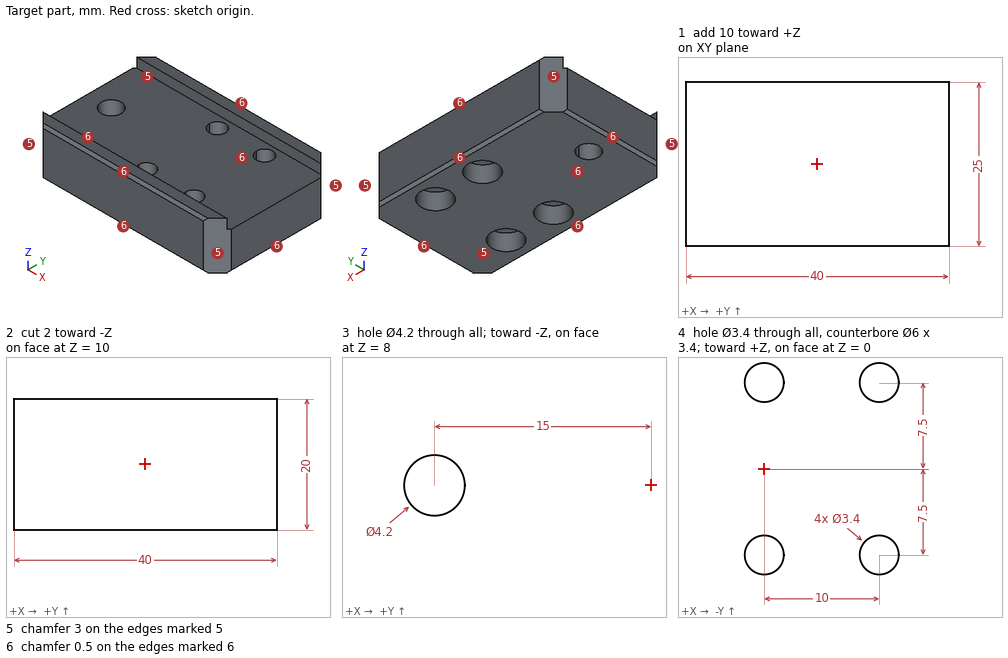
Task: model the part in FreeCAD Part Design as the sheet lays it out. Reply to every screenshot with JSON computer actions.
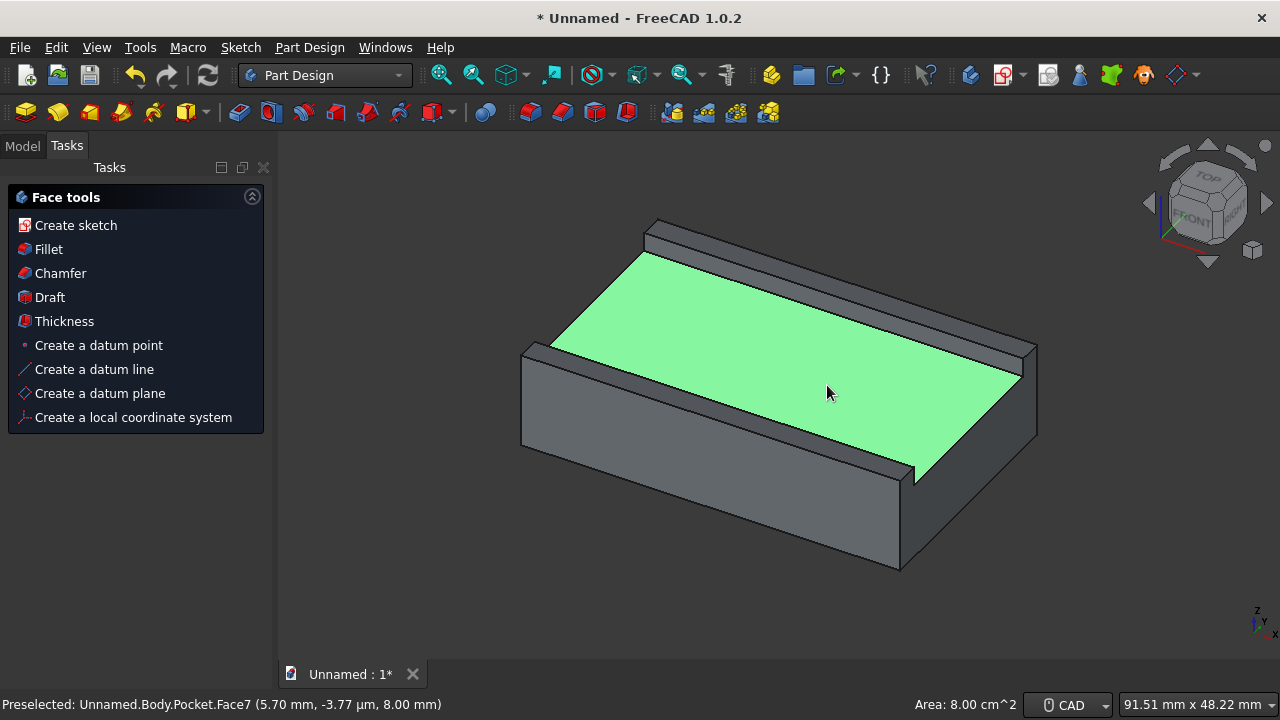
{"action": "left_click", "coordinate": [1004, 76]}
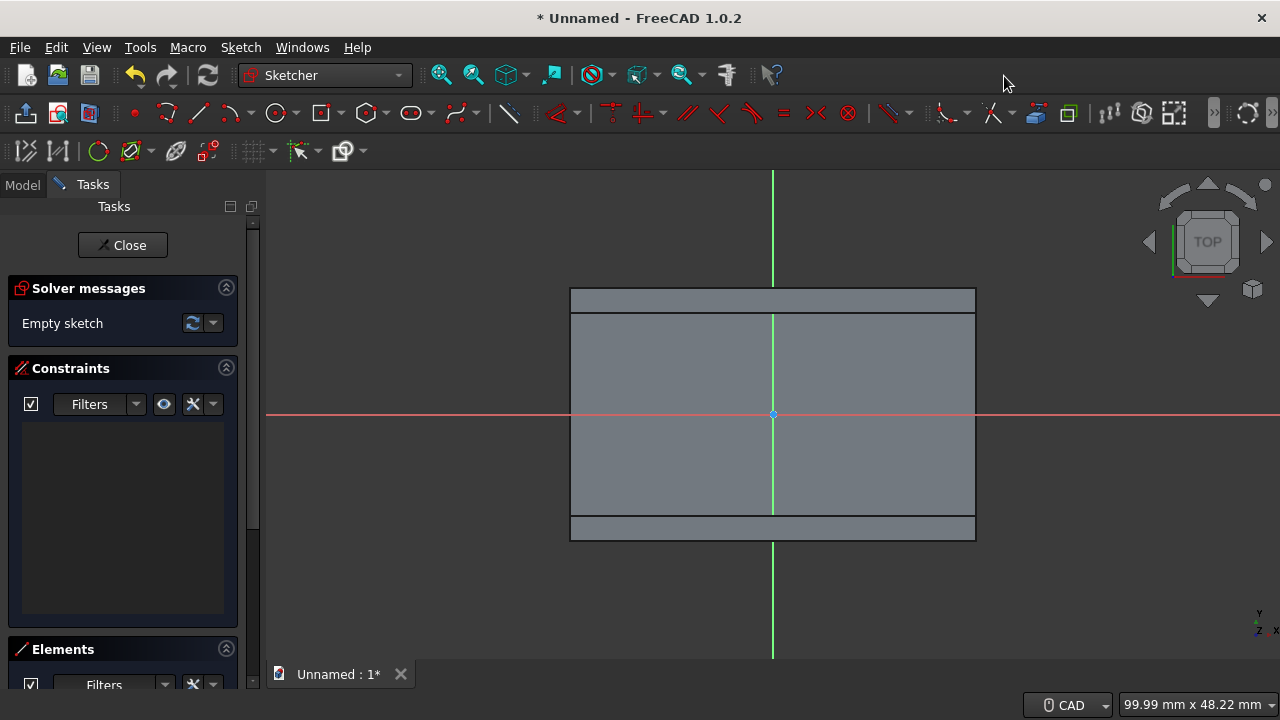
{"action": "left_click", "coordinate": [90, 114]}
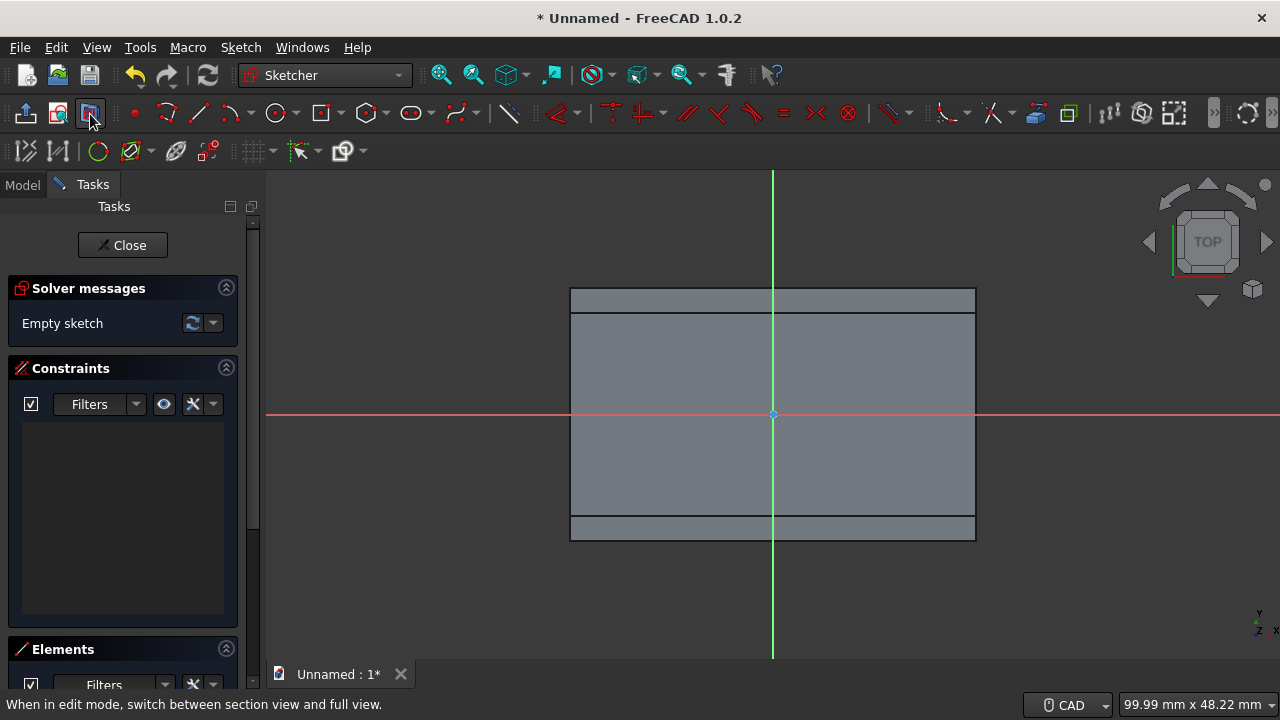
{"action": "scroll", "coordinate": [608, 414], "scroll_direction": "up", "scroll_amount": 10}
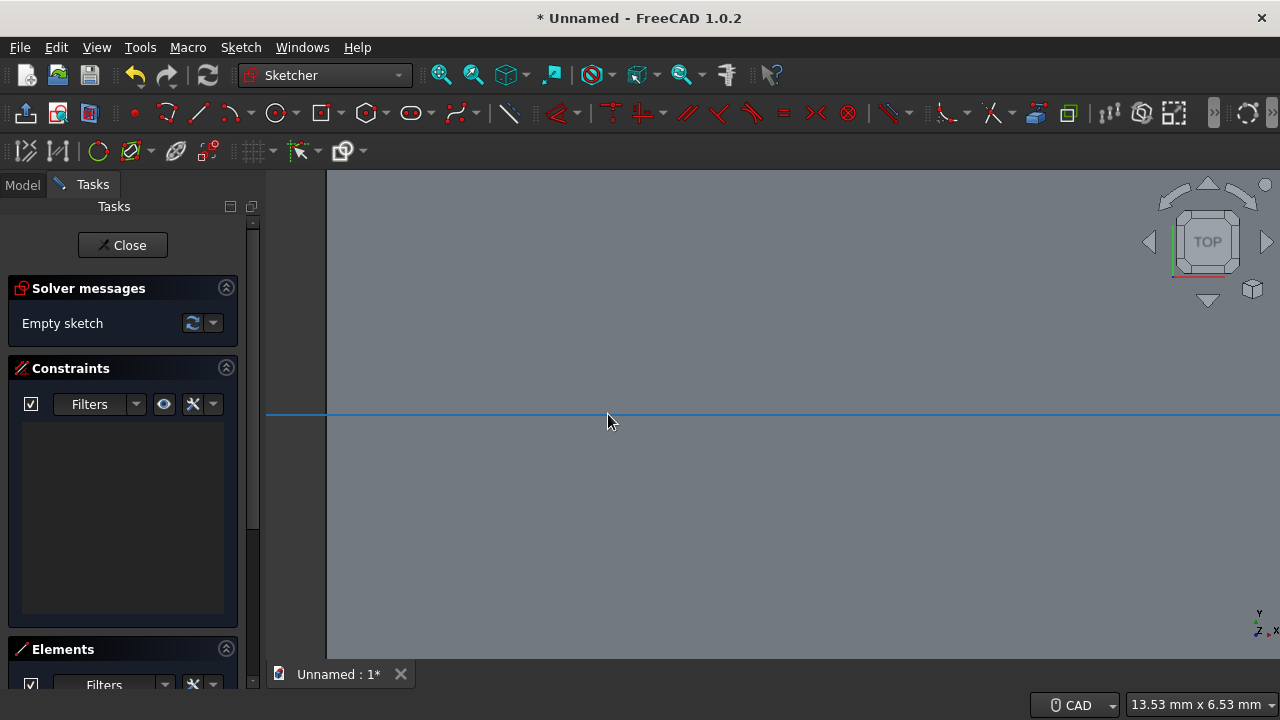
{"action": "left_click", "coordinate": [276, 114]}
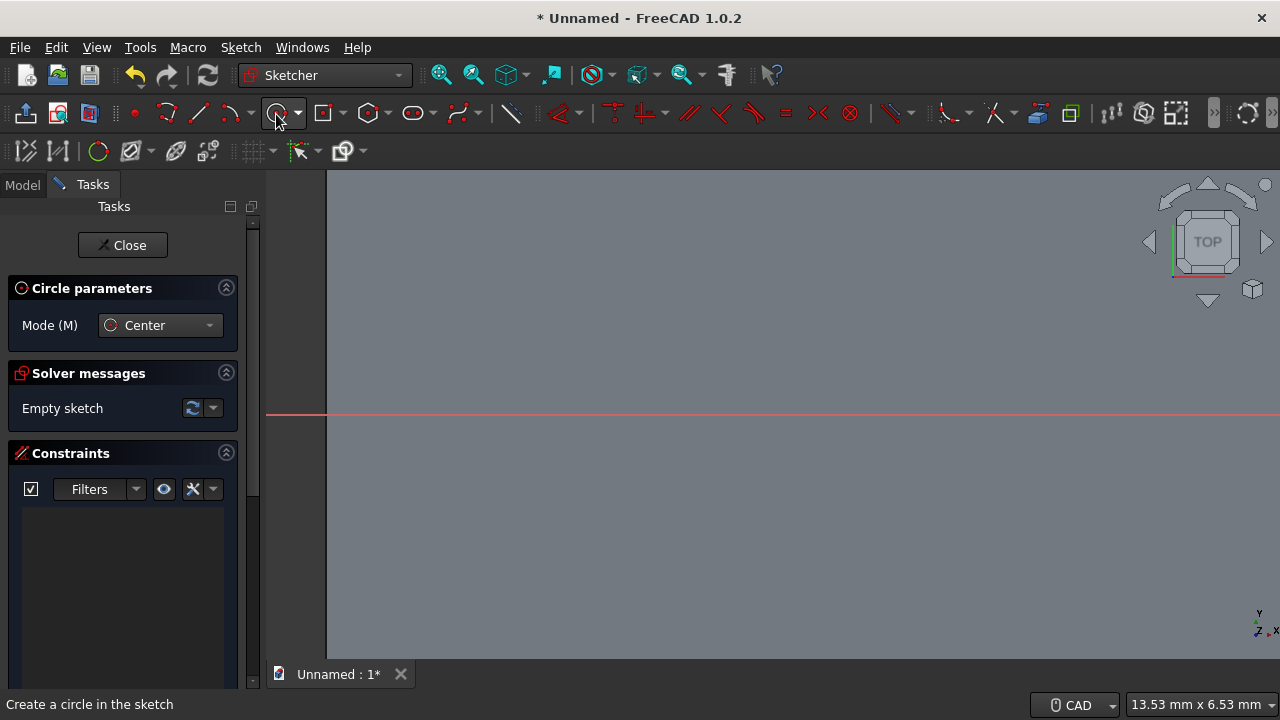
{"action": "left_click", "coordinate": [701, 414]}
{"action": "left_click", "coordinate": [812, 303]}
{"action": "key", "text": "Escape"}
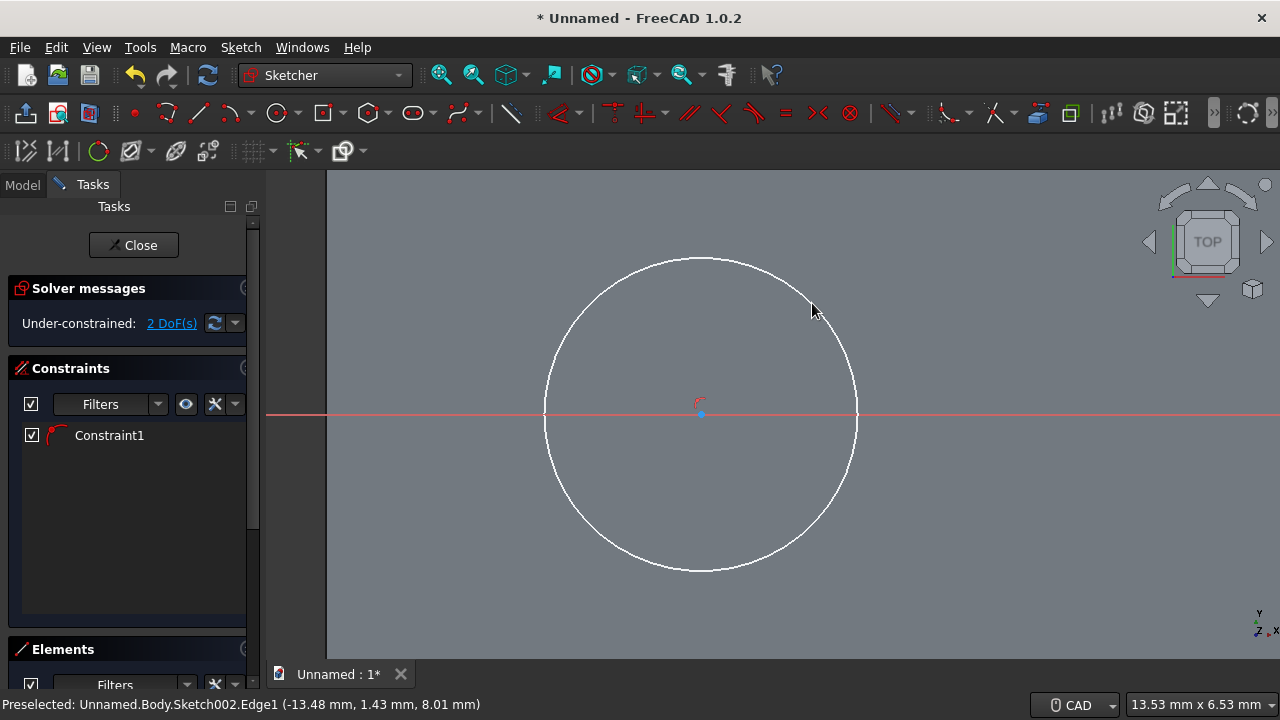
{"action": "left_click", "coordinate": [558, 114]}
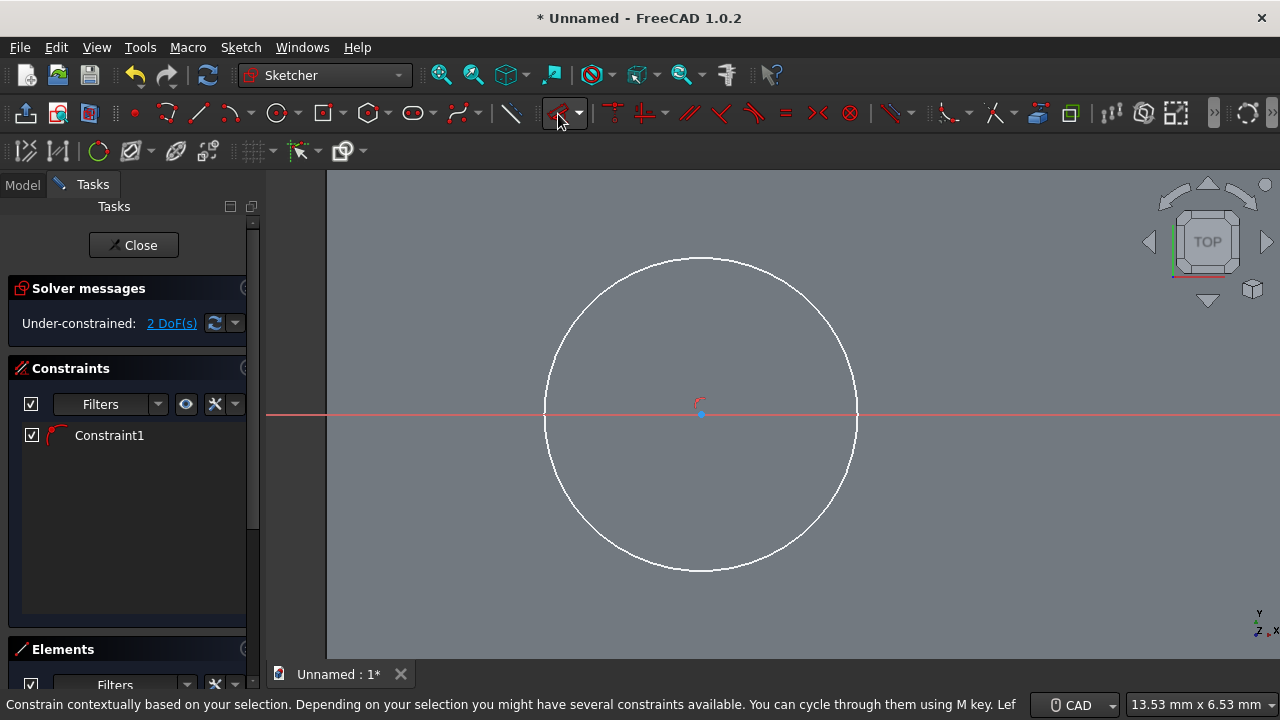
{"action": "left_click", "coordinate": [811, 303]}
{"action": "left_click", "coordinate": [833, 280]}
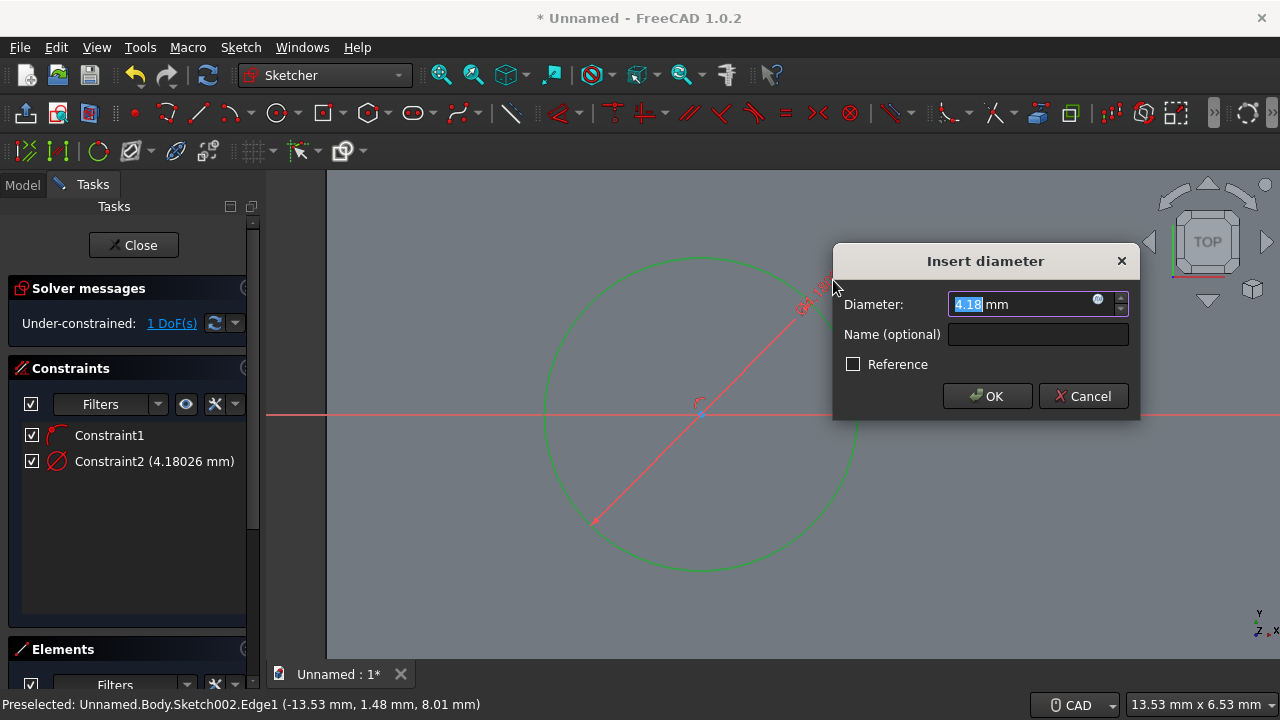
{"action": "type", "text": "4.2"}
{"action": "key", "text": "Return"}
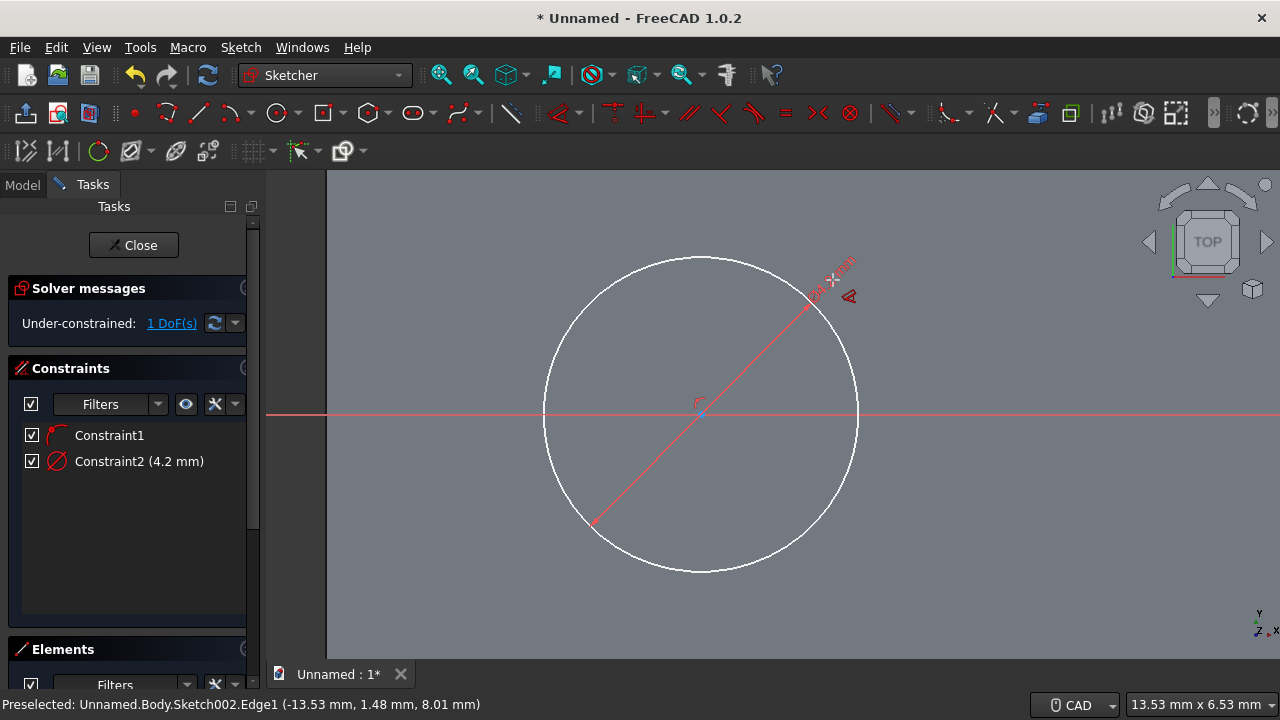
{"action": "left_click", "coordinate": [701, 414]}
{"action": "left_click", "coordinate": [908, 448]}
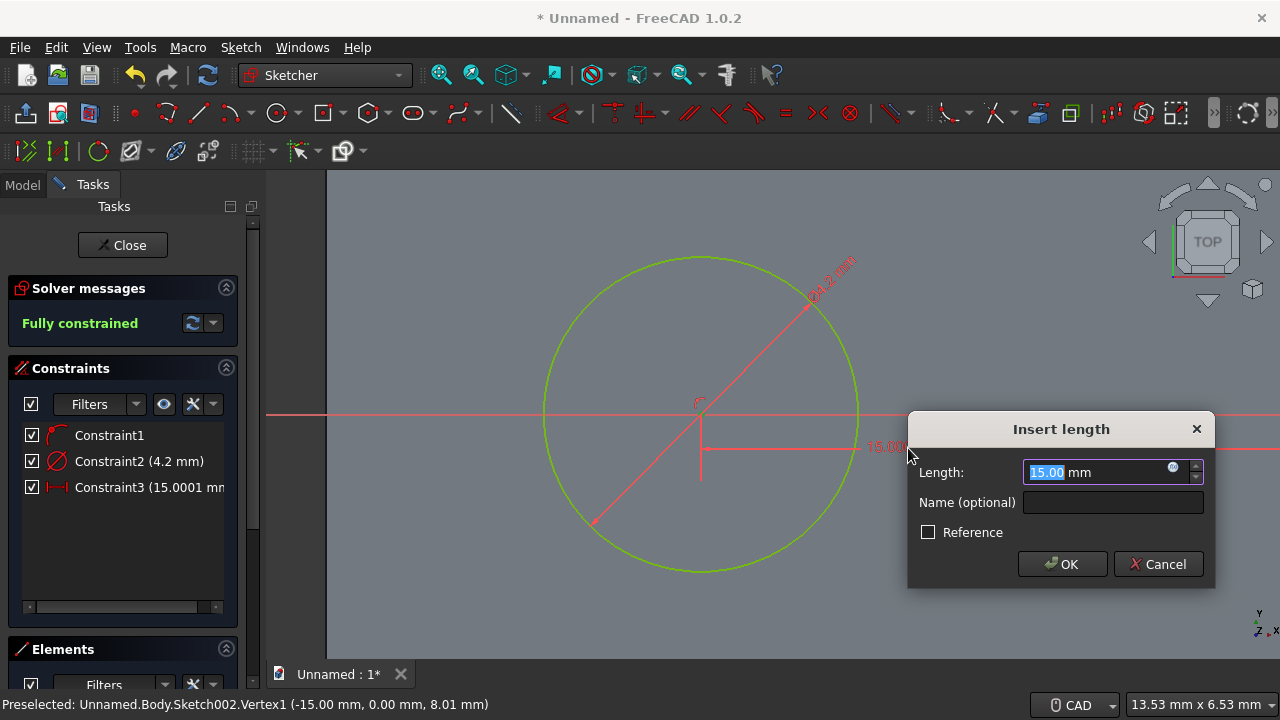
{"action": "type", "text": "15"}
{"action": "key", "text": "Return"}
{"action": "key", "text": "Escape"}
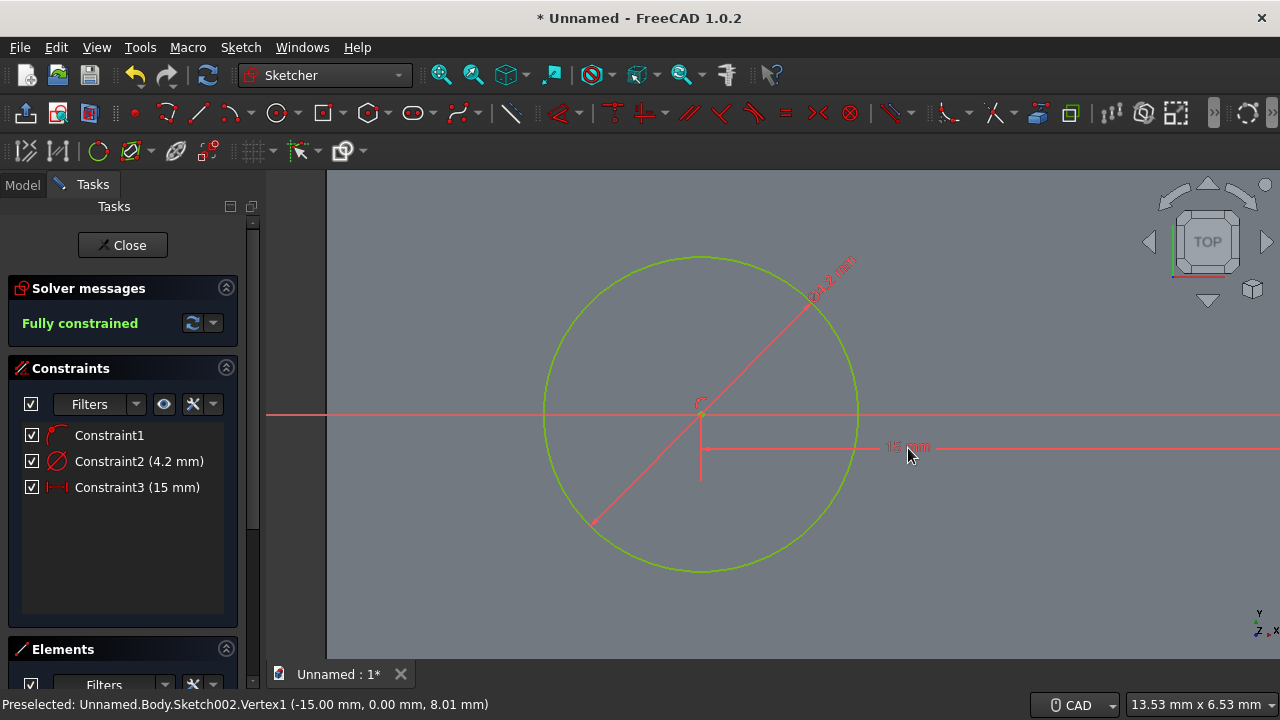
{"action": "left_click", "coordinate": [123, 245]}